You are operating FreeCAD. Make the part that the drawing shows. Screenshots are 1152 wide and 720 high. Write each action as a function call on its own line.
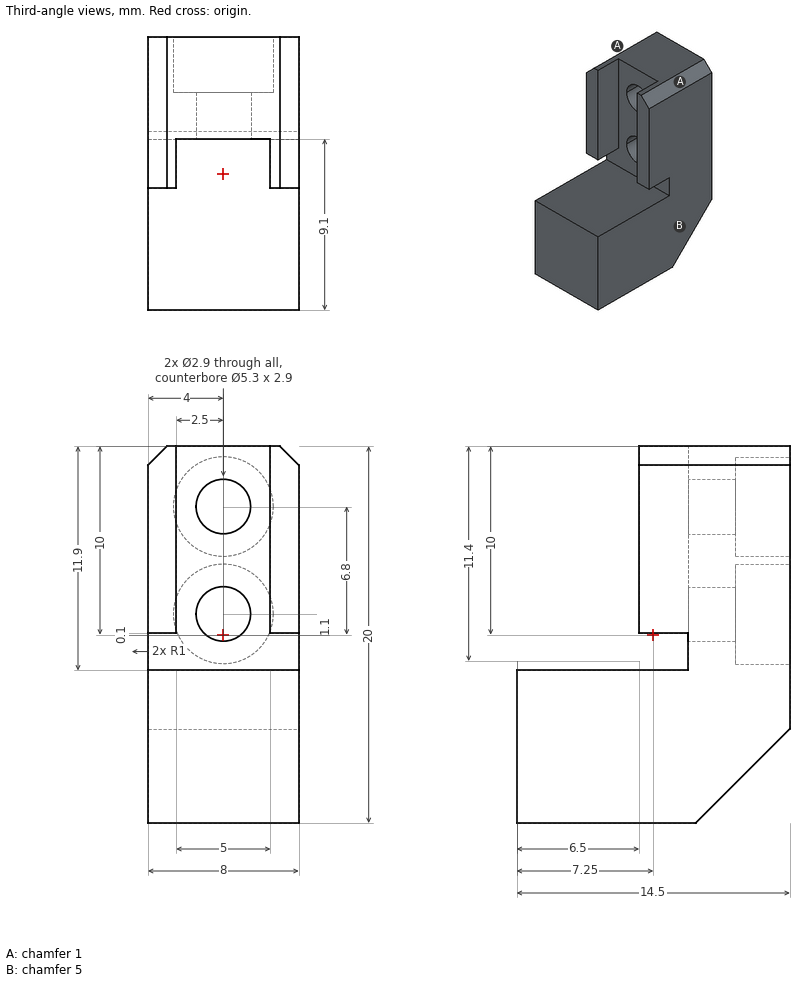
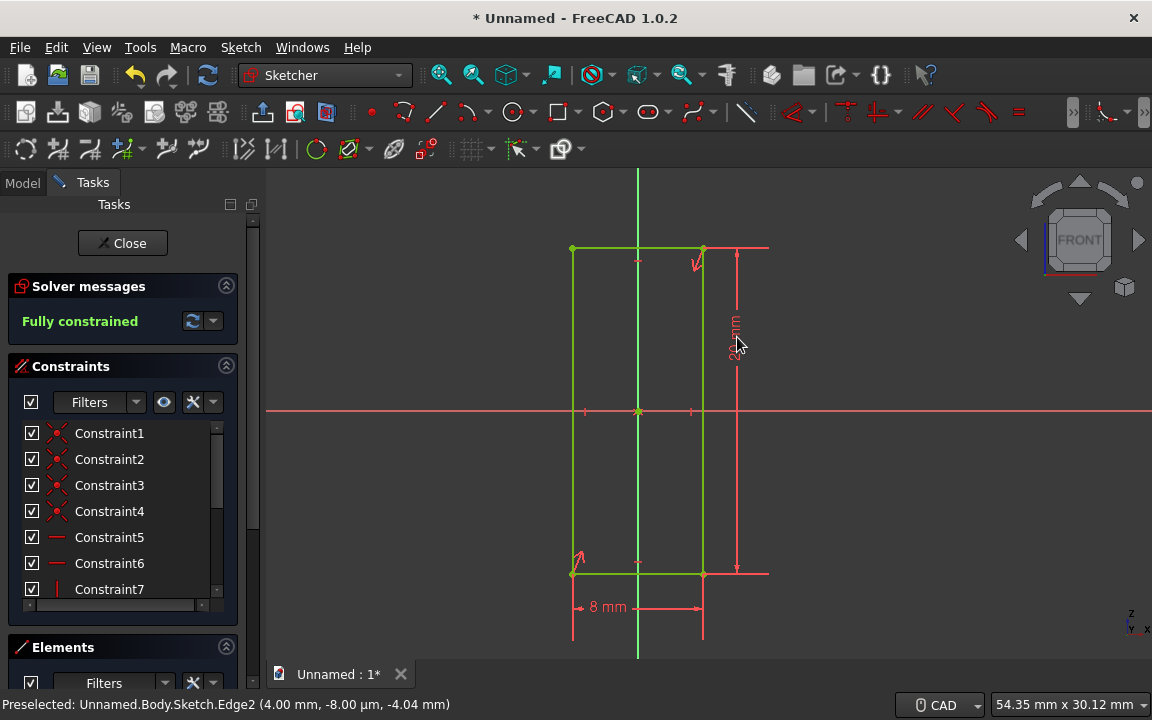
click(123, 243)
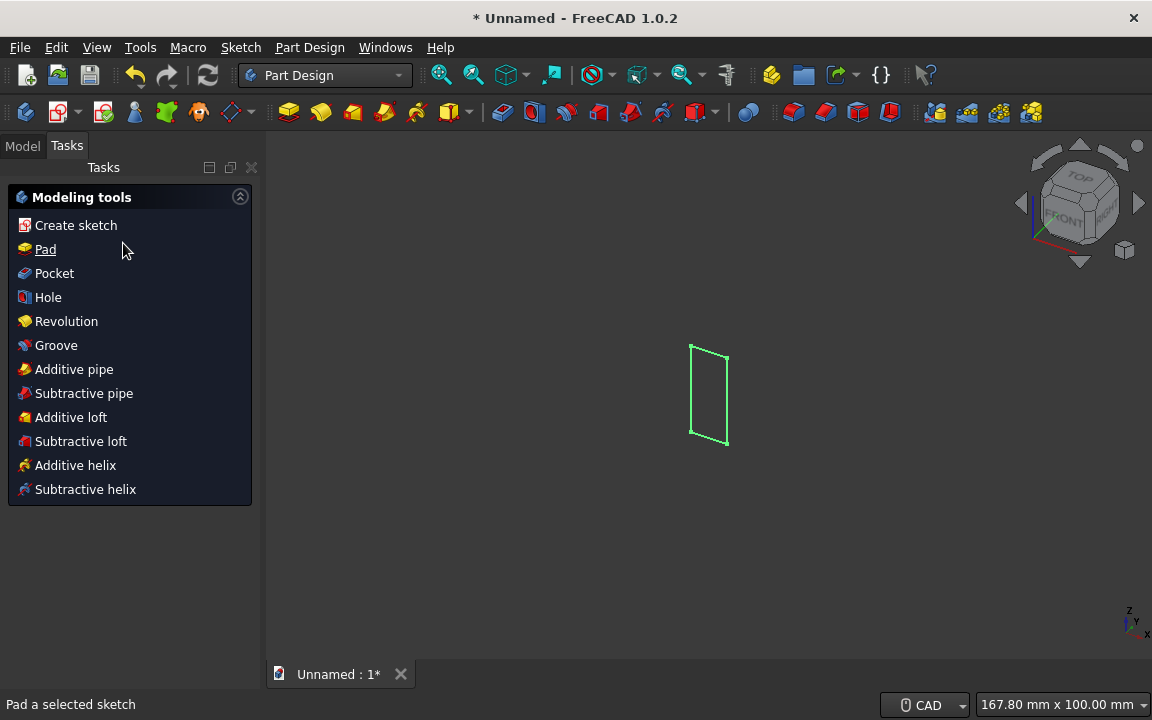
click(290, 112)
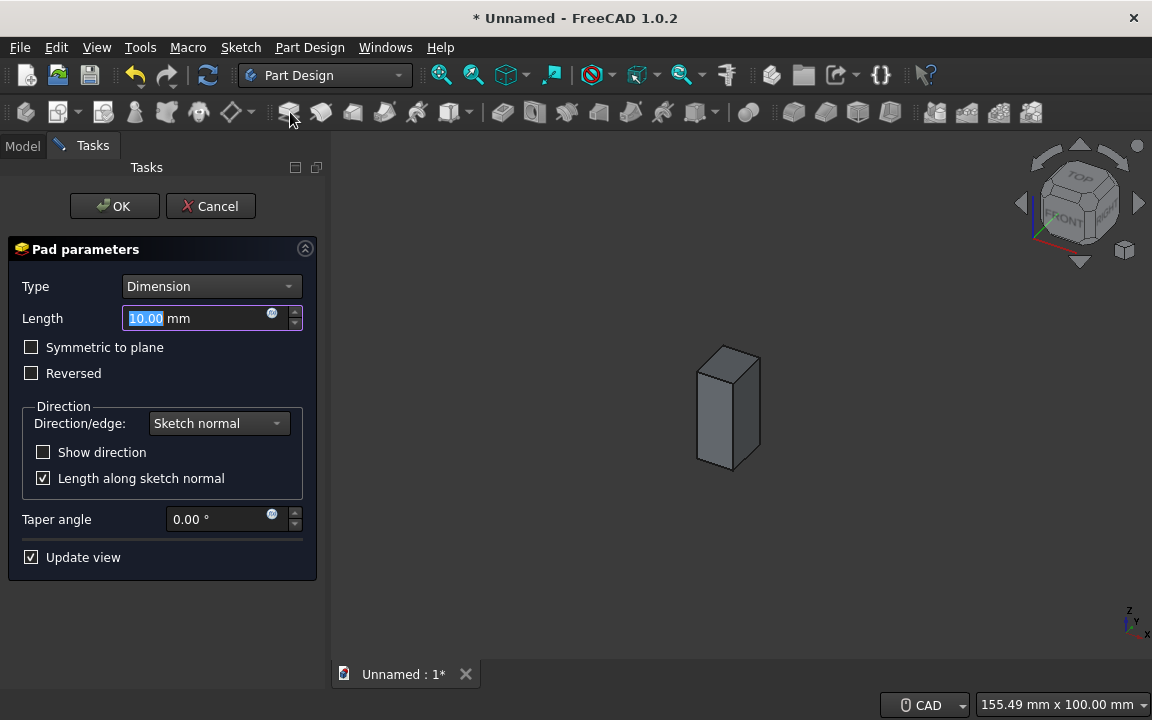
text(14.5)
key(Tab)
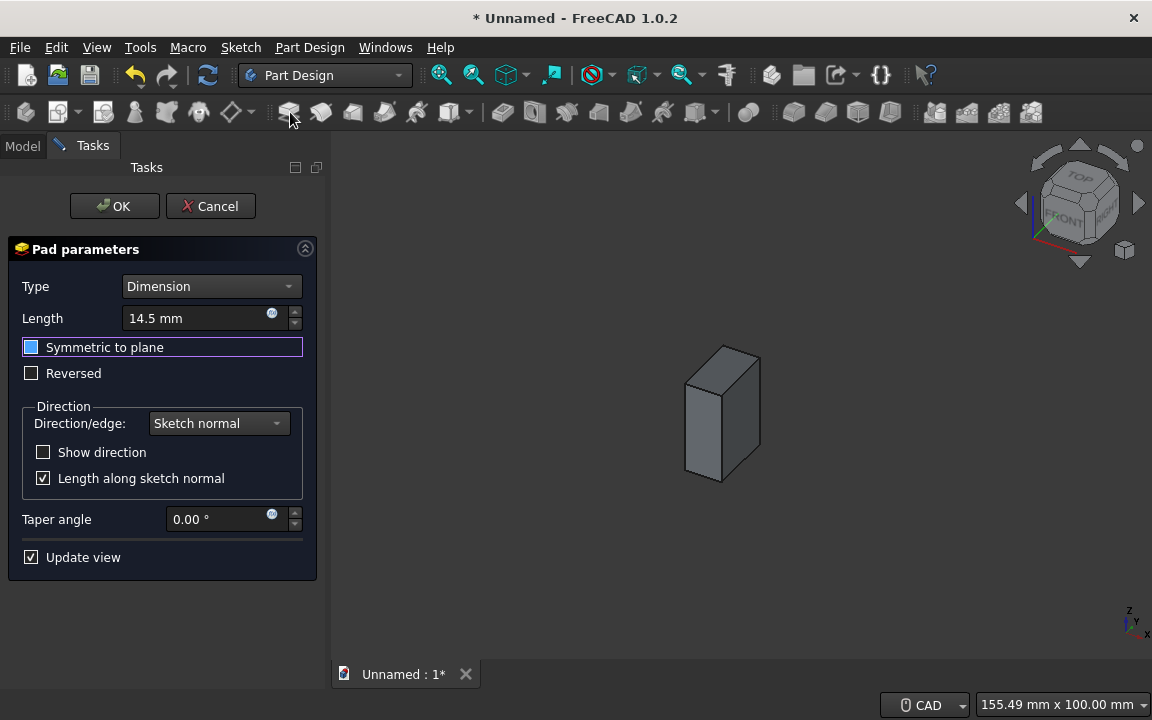
click(30, 347)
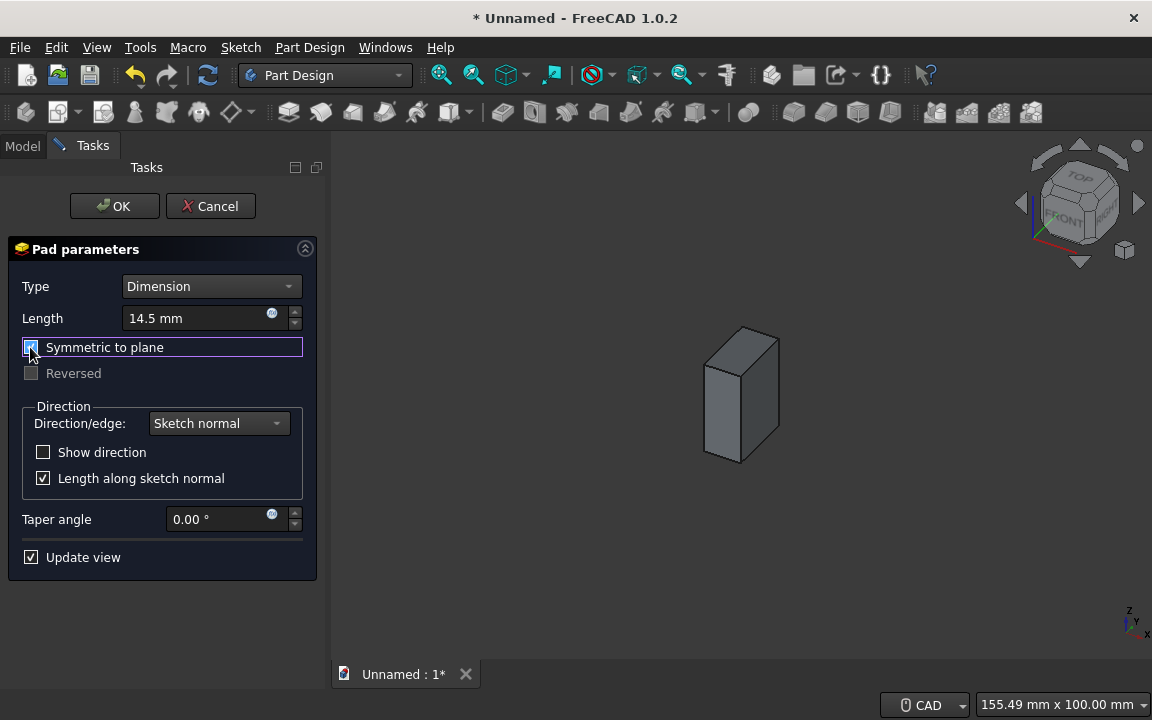
click(115, 206)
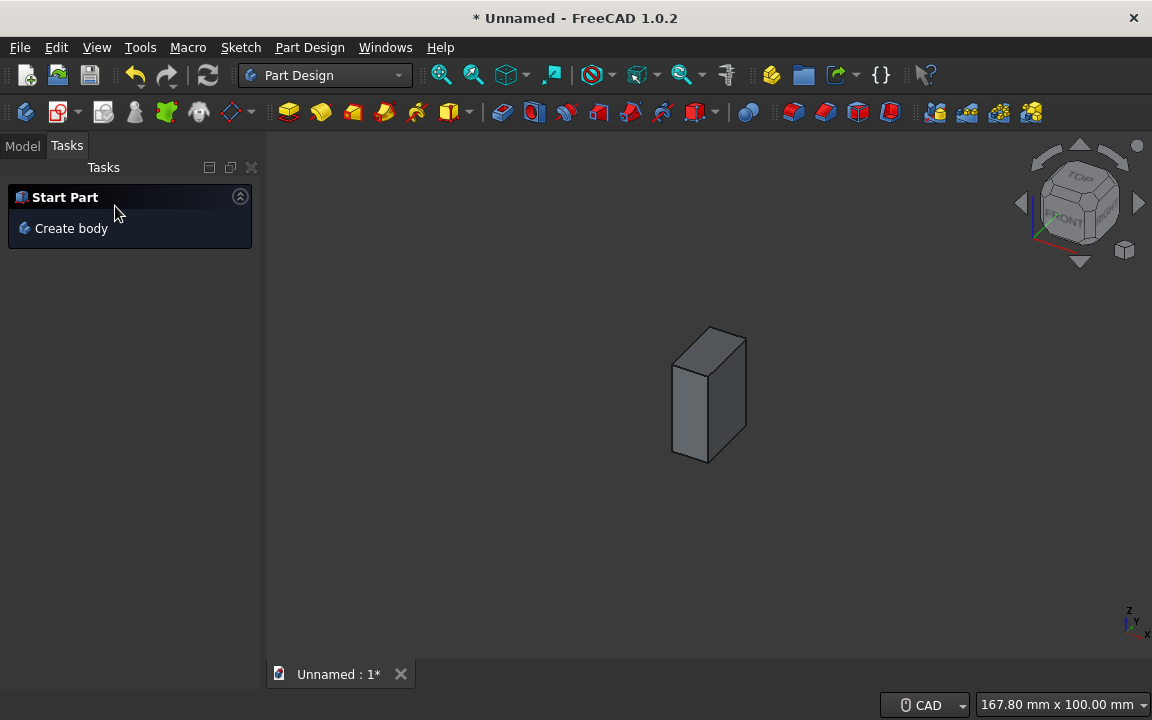
key(v)
key(f)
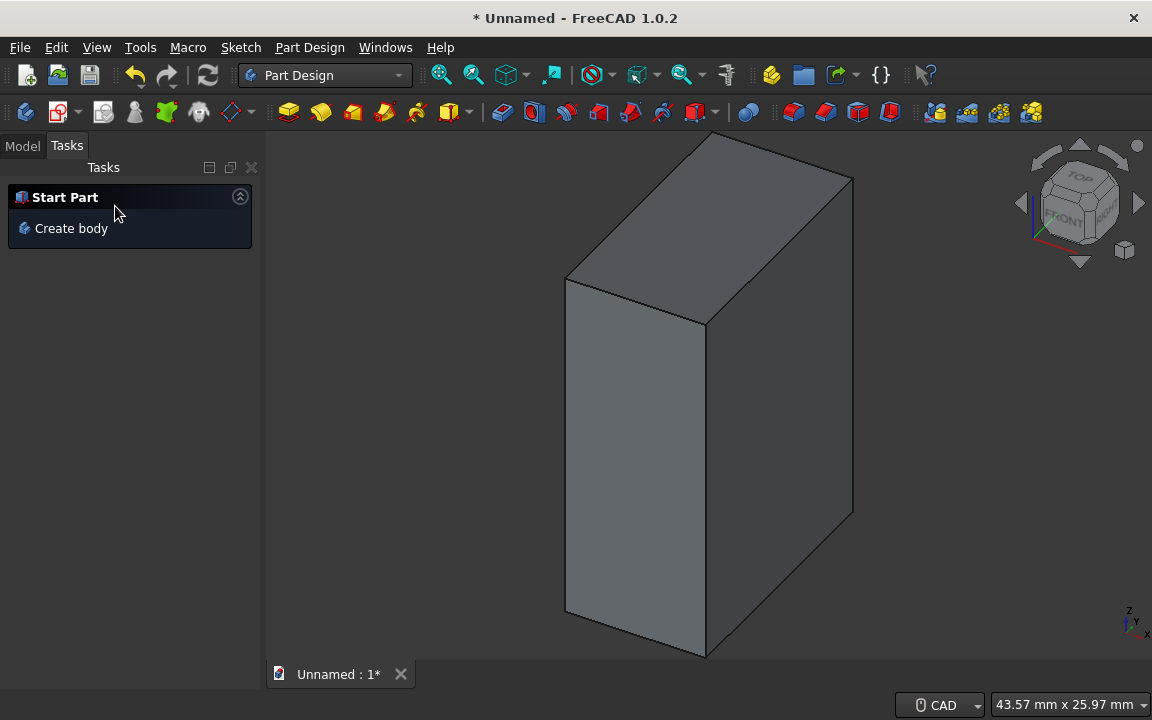
click(635, 372)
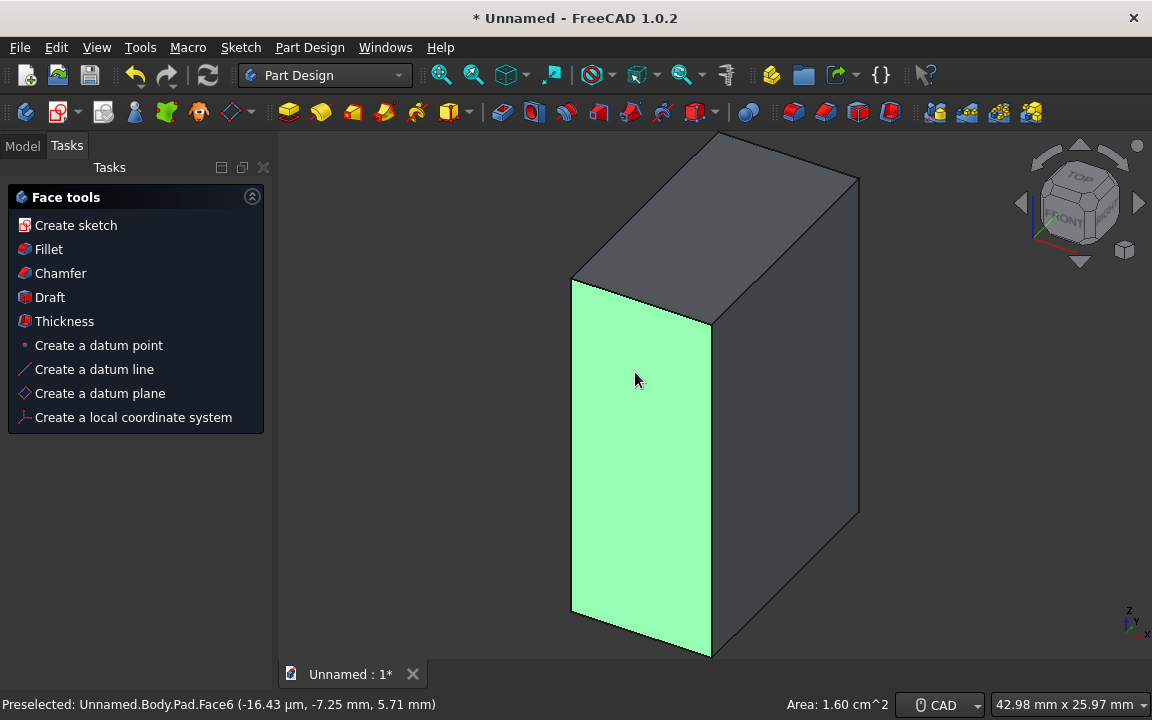
click(58, 112)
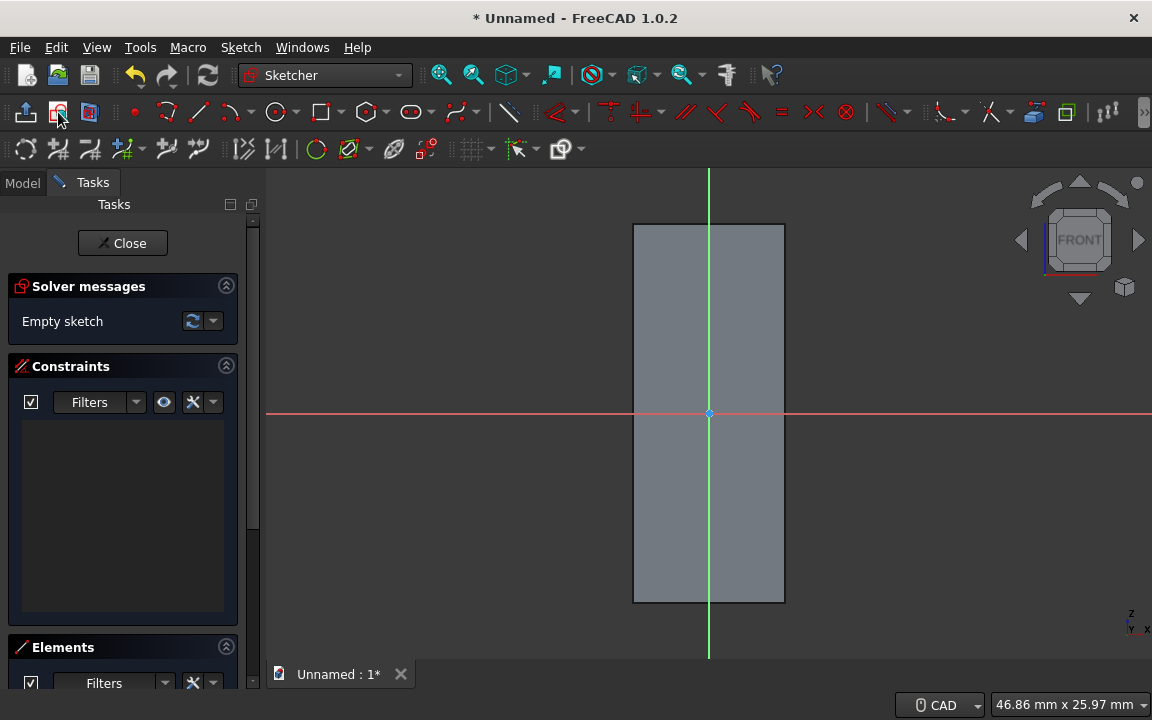
scroll(848, 196, up, 2)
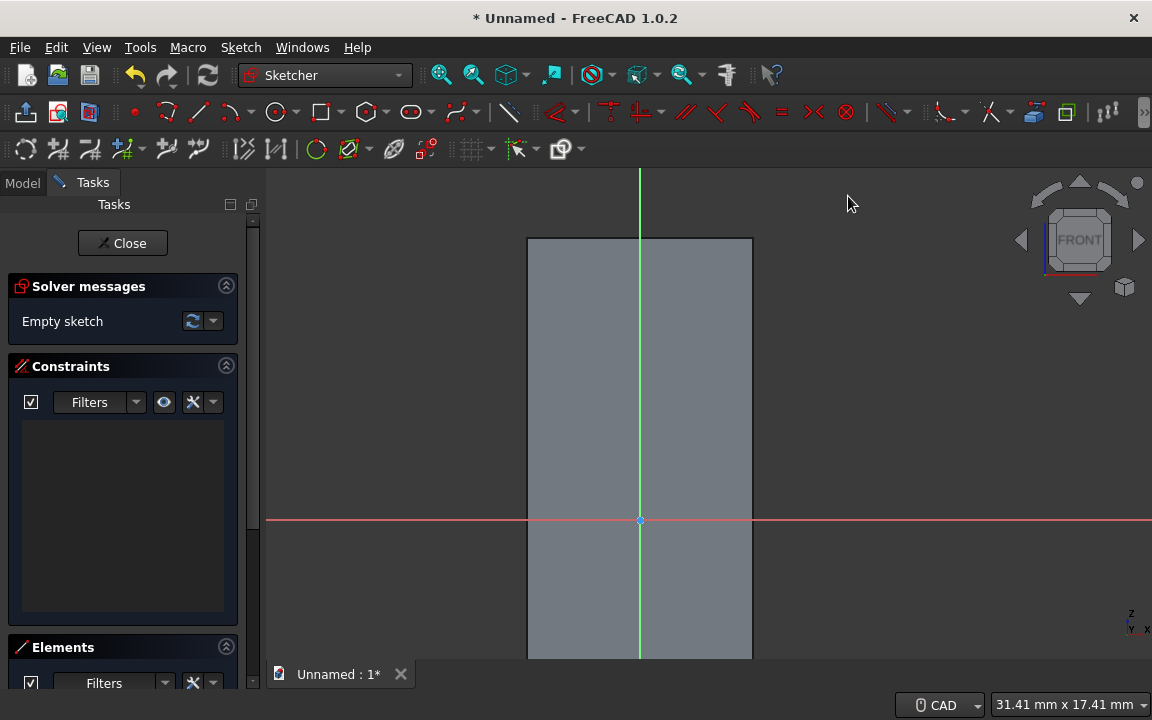
key(g)
key(r)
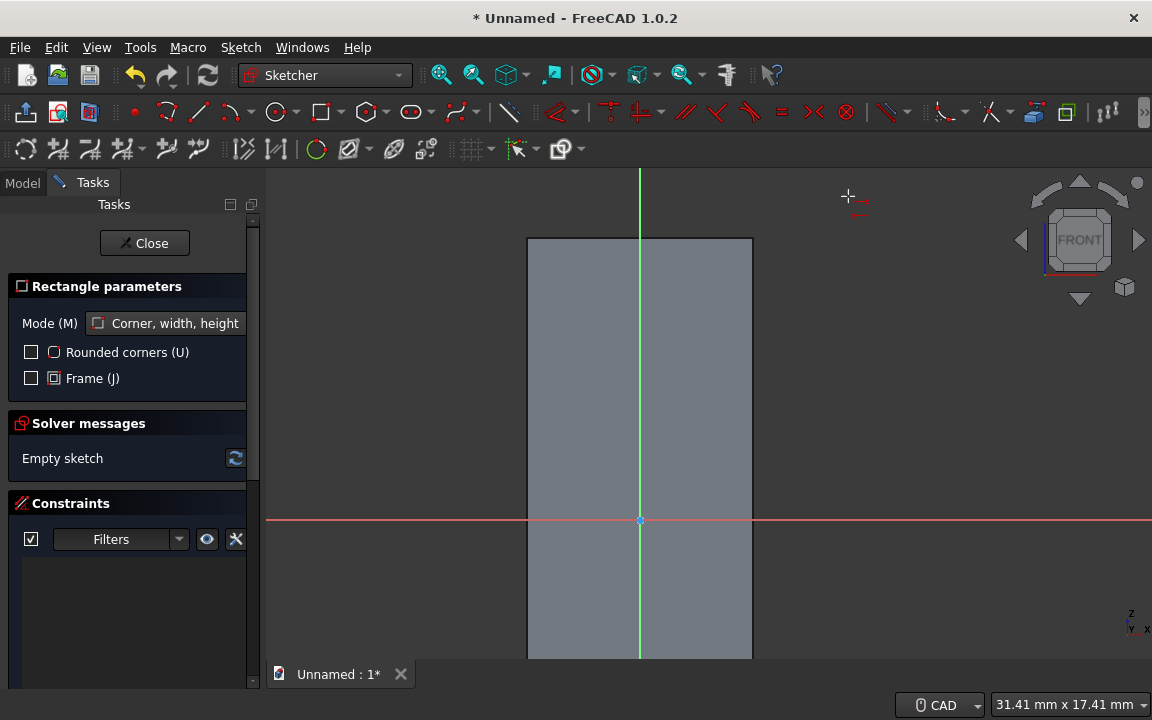
click(570, 238)
click(711, 574)
key(Escape)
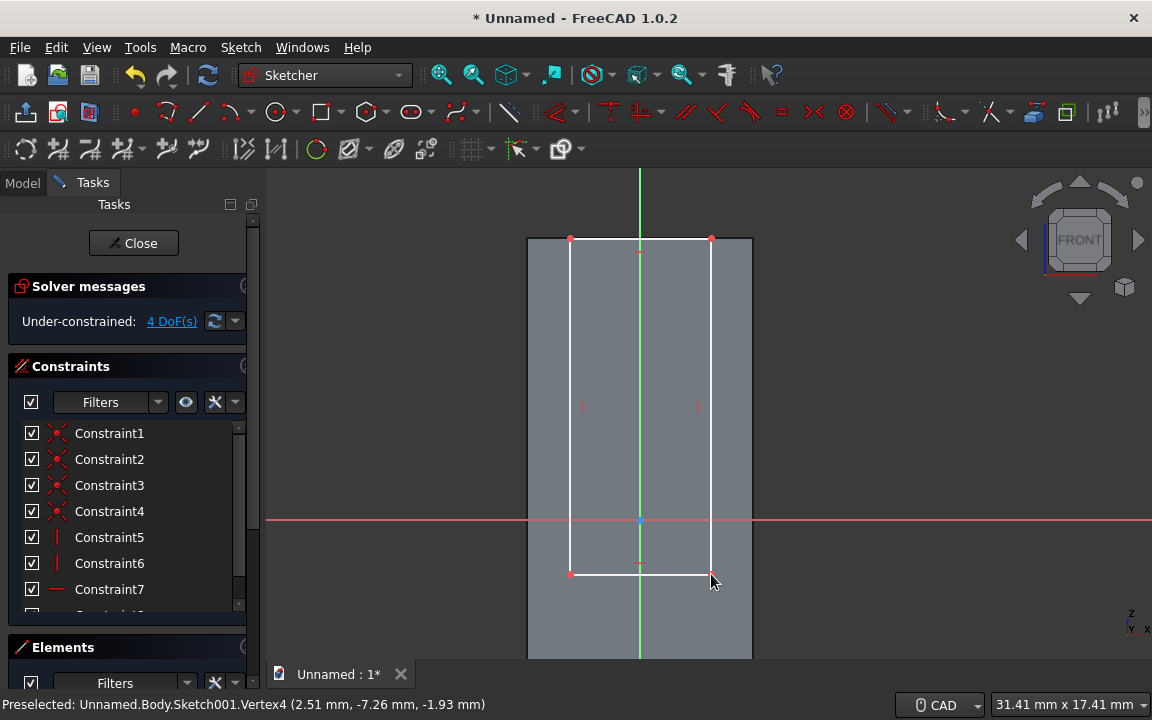
click(556, 112)